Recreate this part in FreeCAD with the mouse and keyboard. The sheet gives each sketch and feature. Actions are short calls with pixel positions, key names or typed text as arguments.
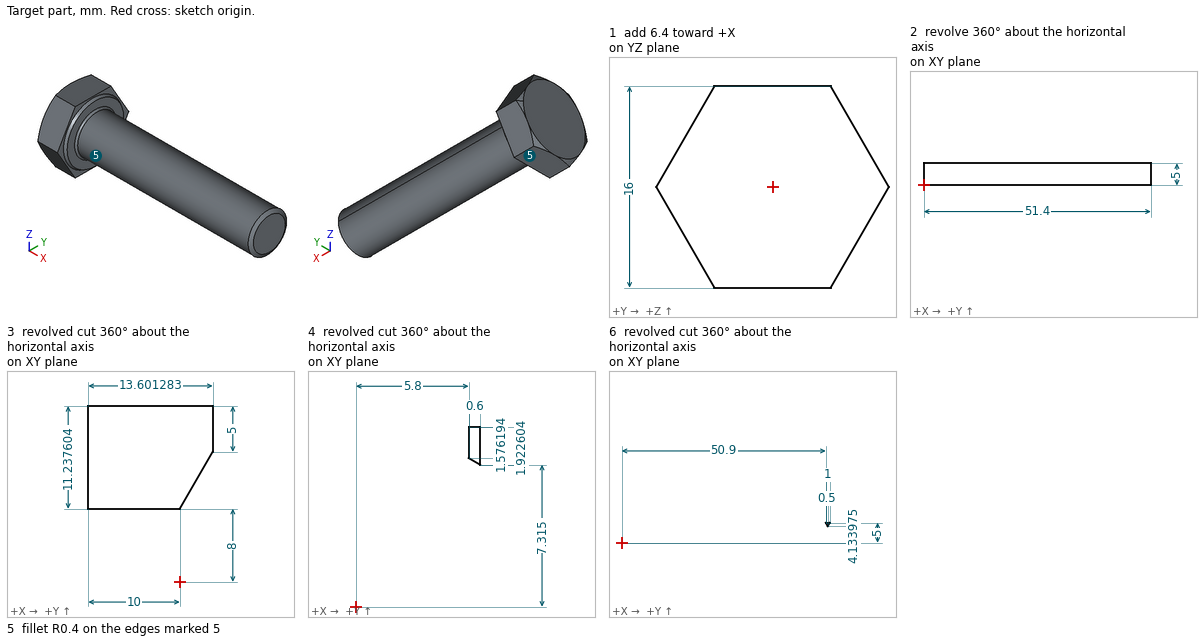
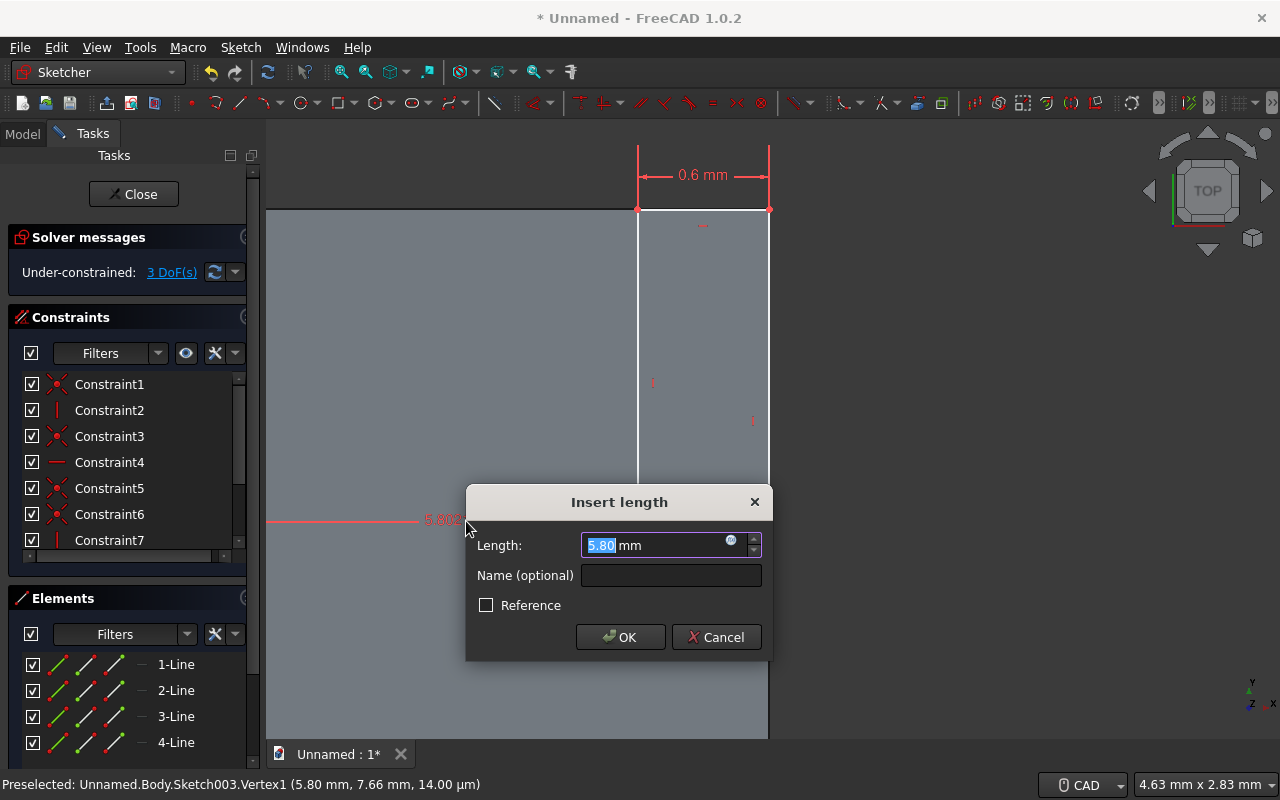
text(5.8)
key(Return)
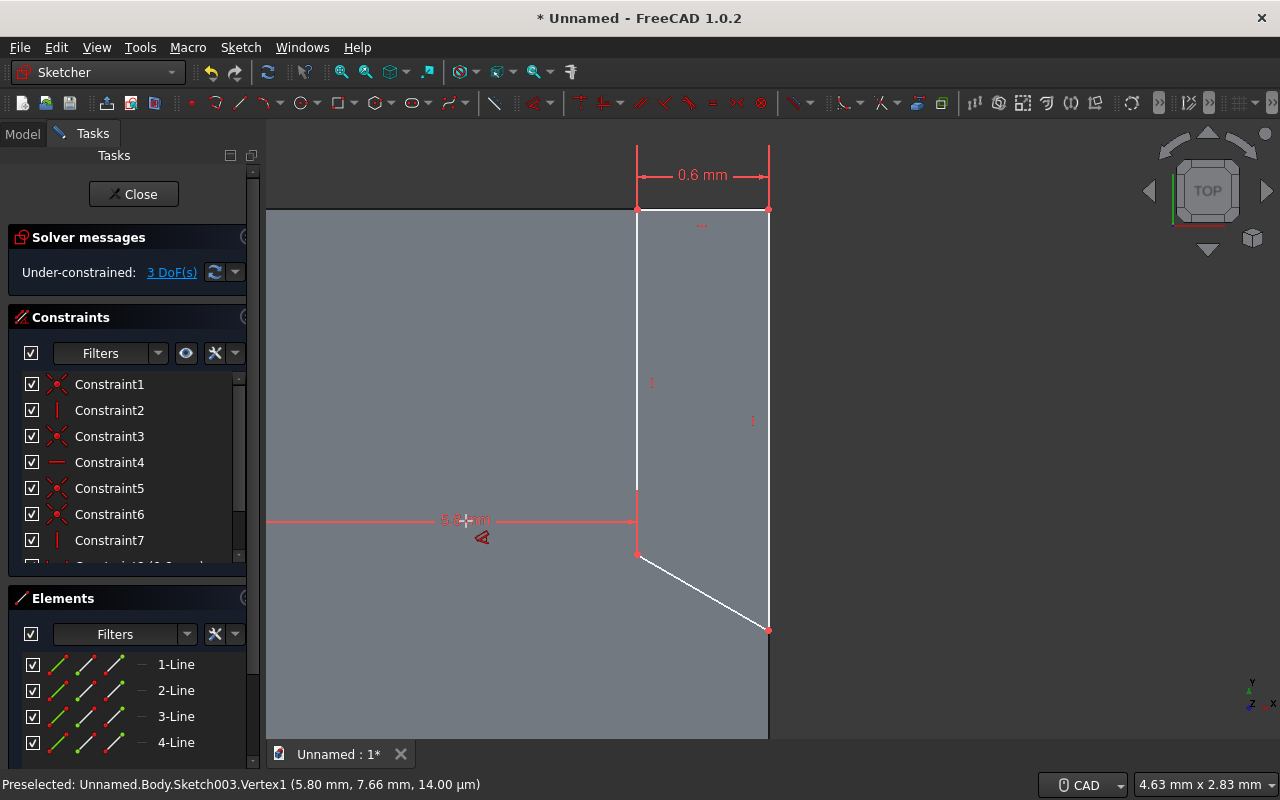
click(769, 631)
click(803, 671)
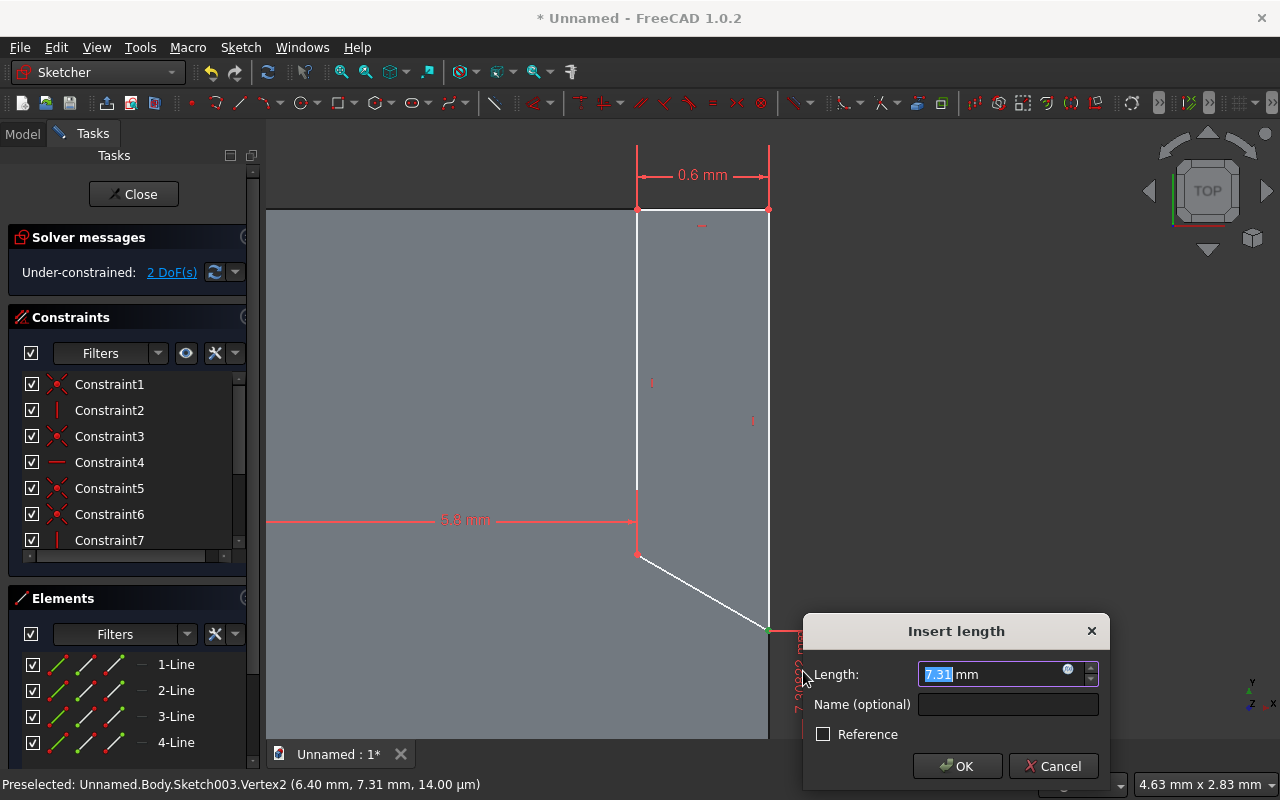
text(7.315)
key(Return)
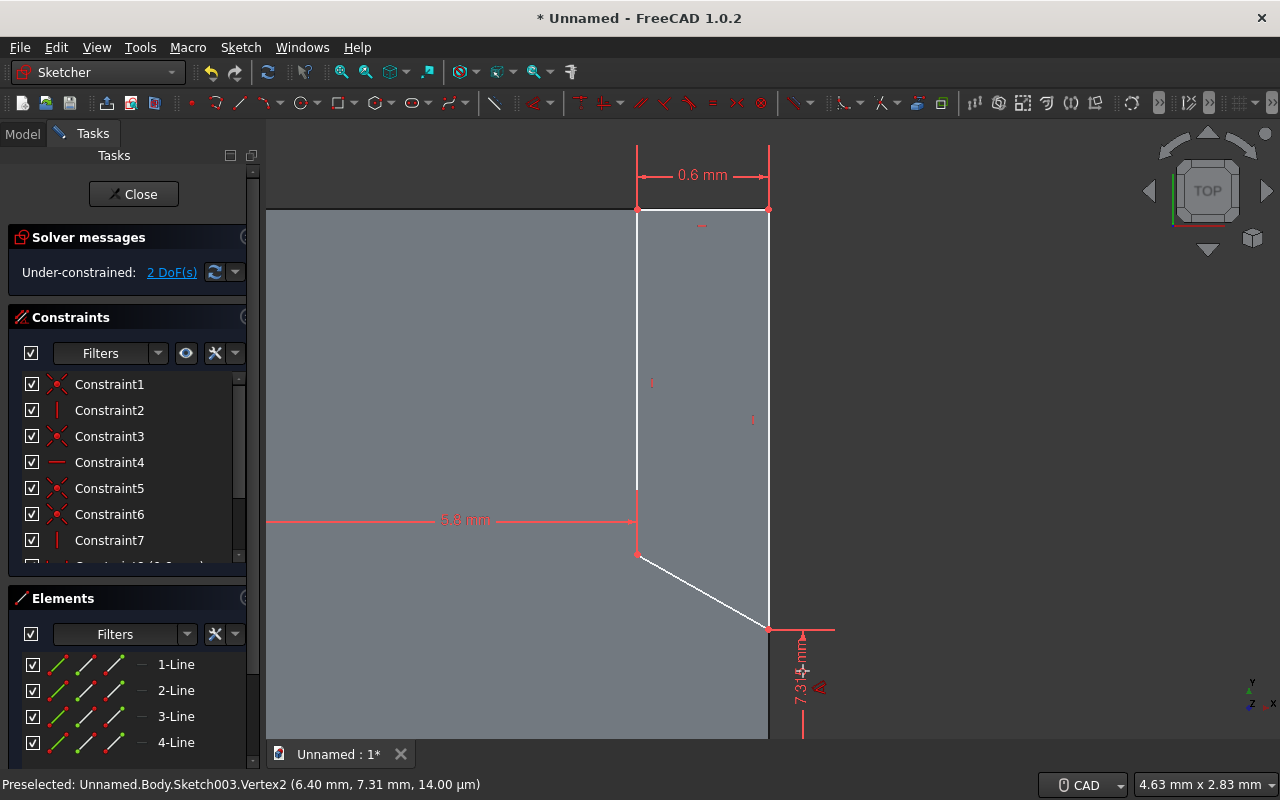
click(769, 504)
click(803, 420)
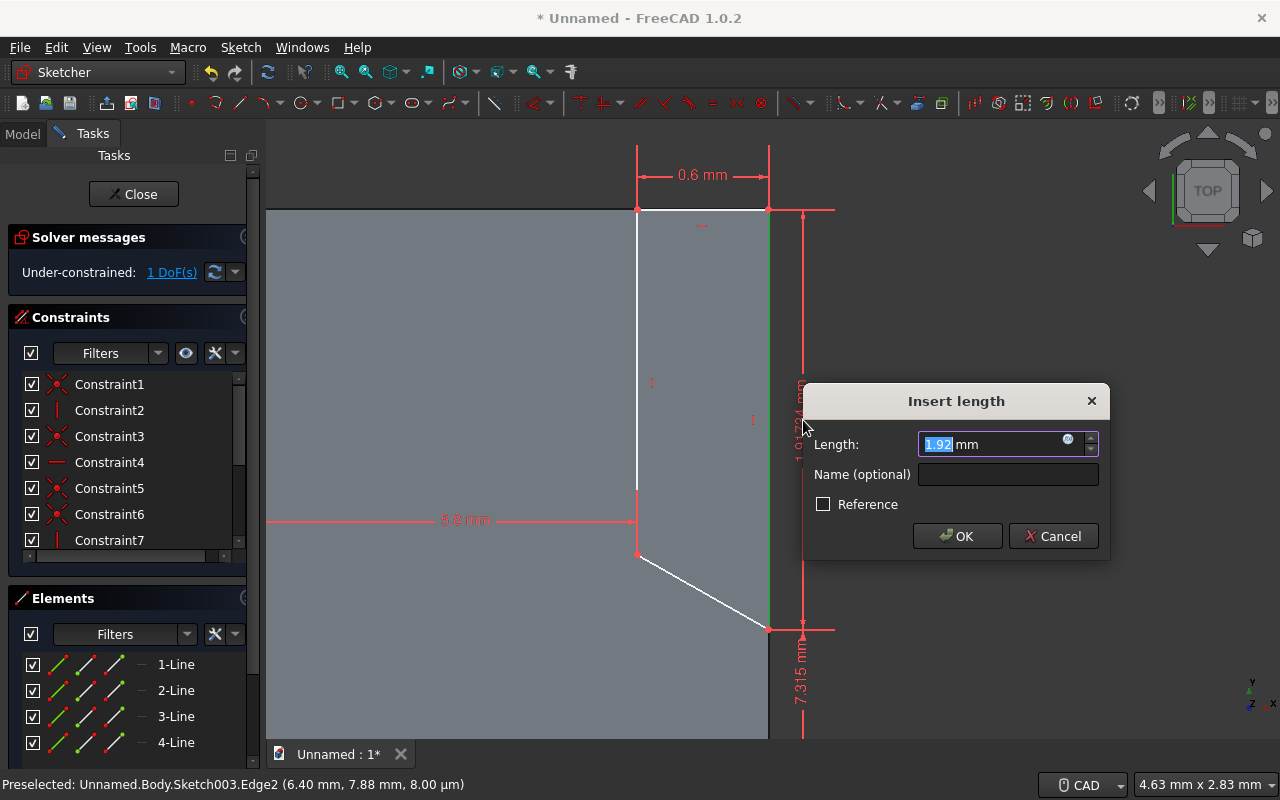
text(1.922604)
key(Return)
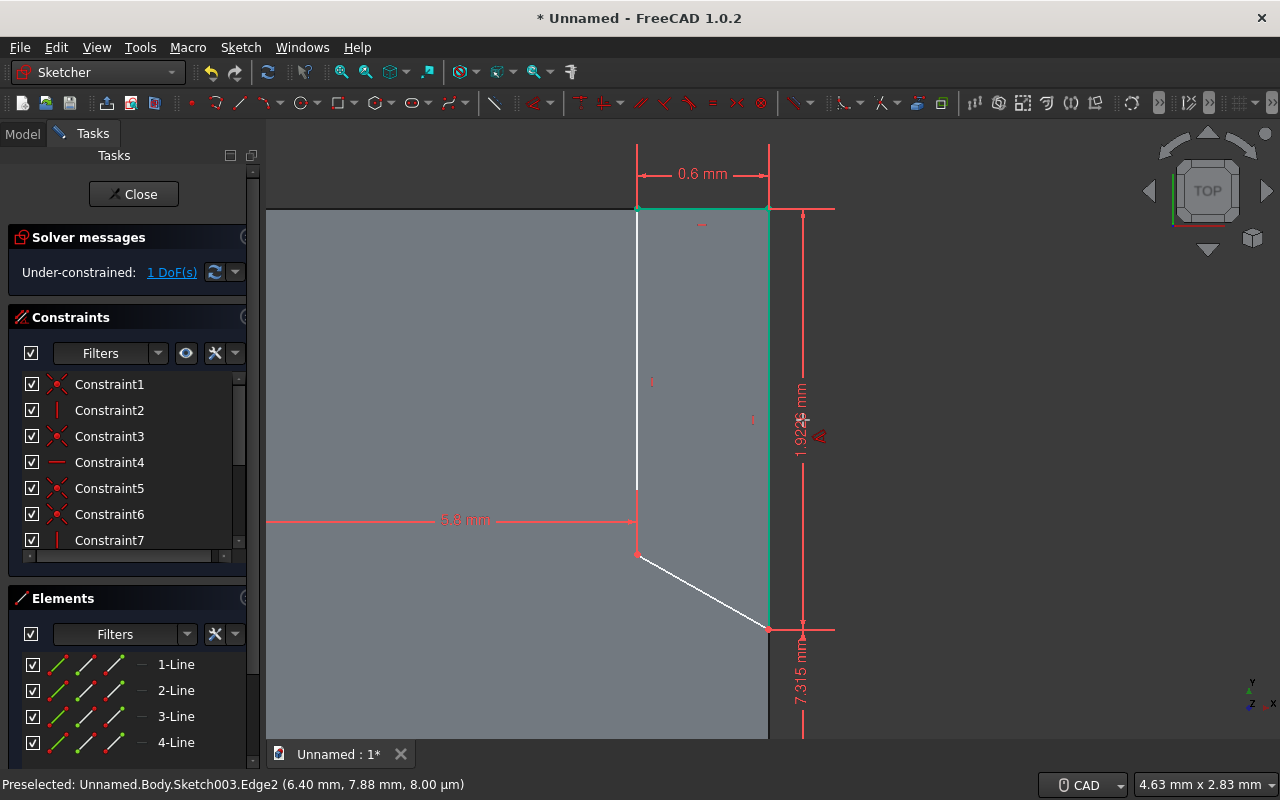
click(637, 313)
click(603, 382)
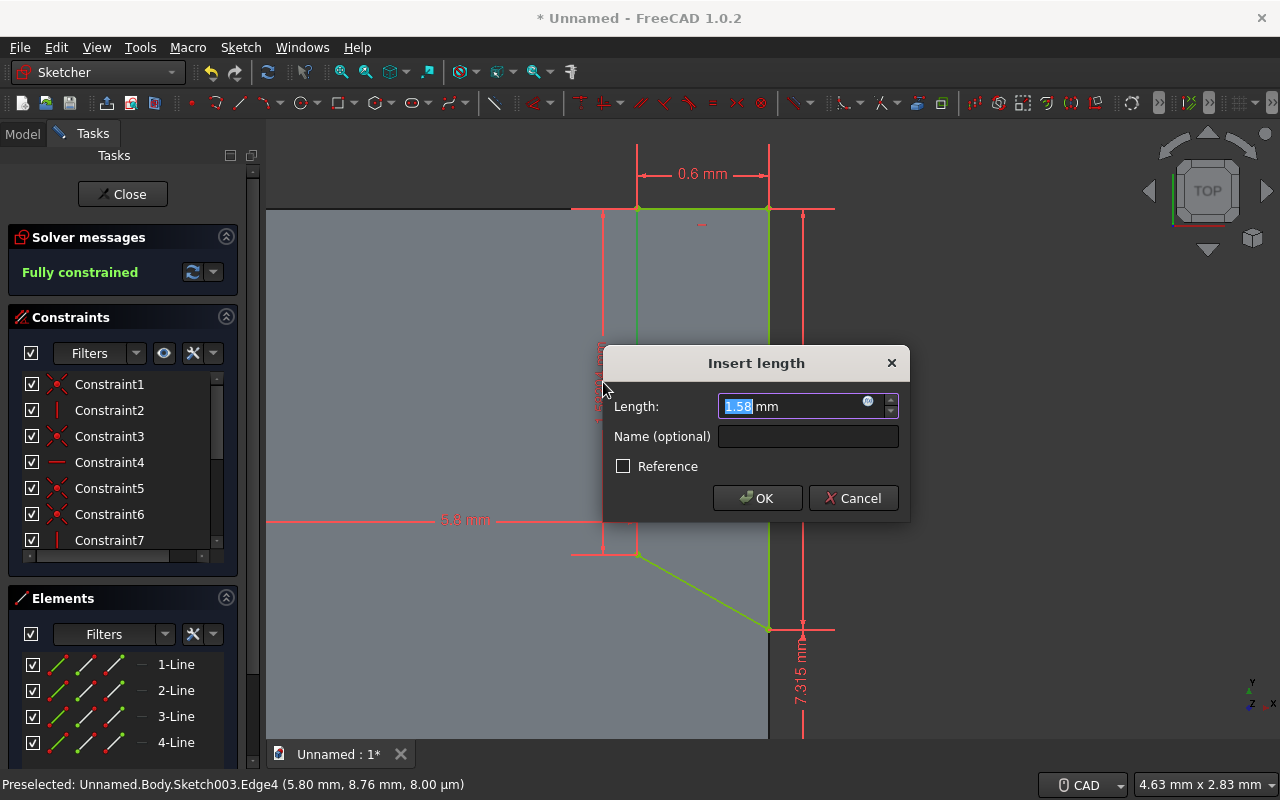
text(1.576194)
key(Return)
key(Escape)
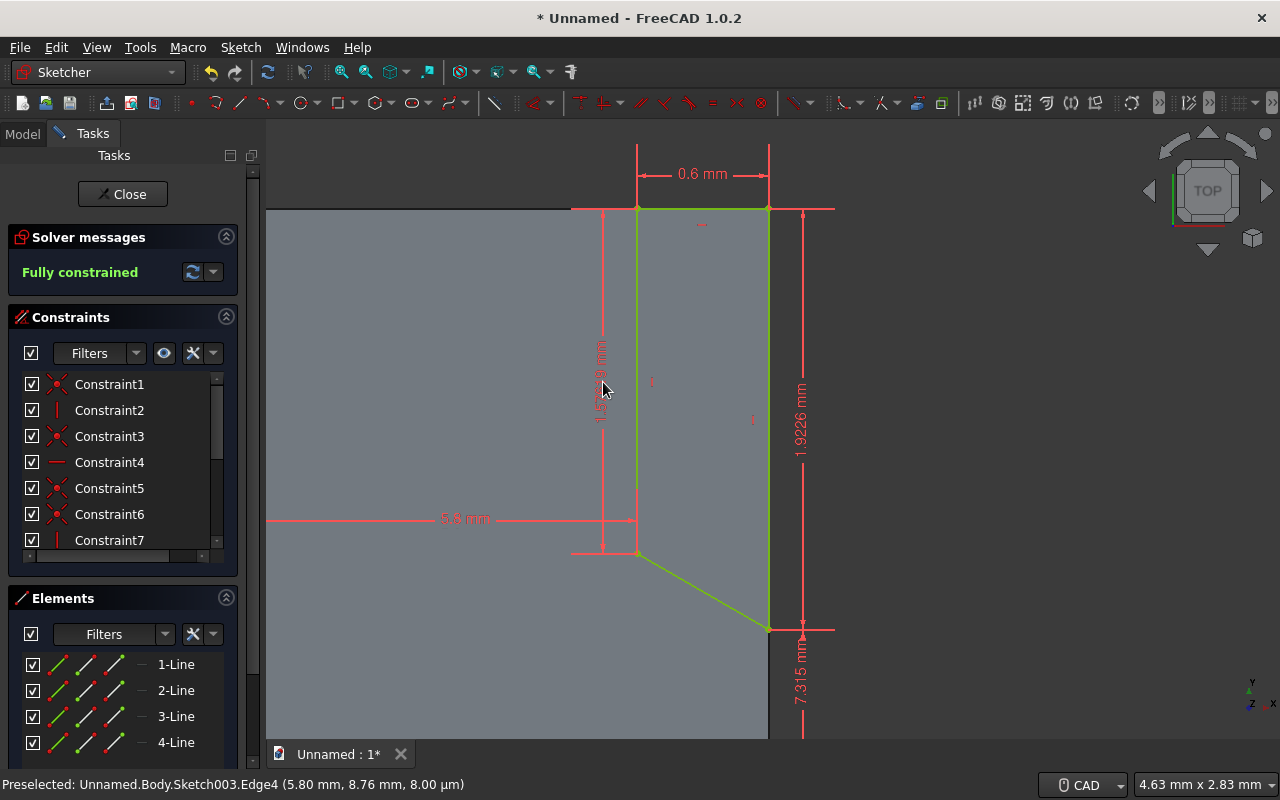
click(123, 194)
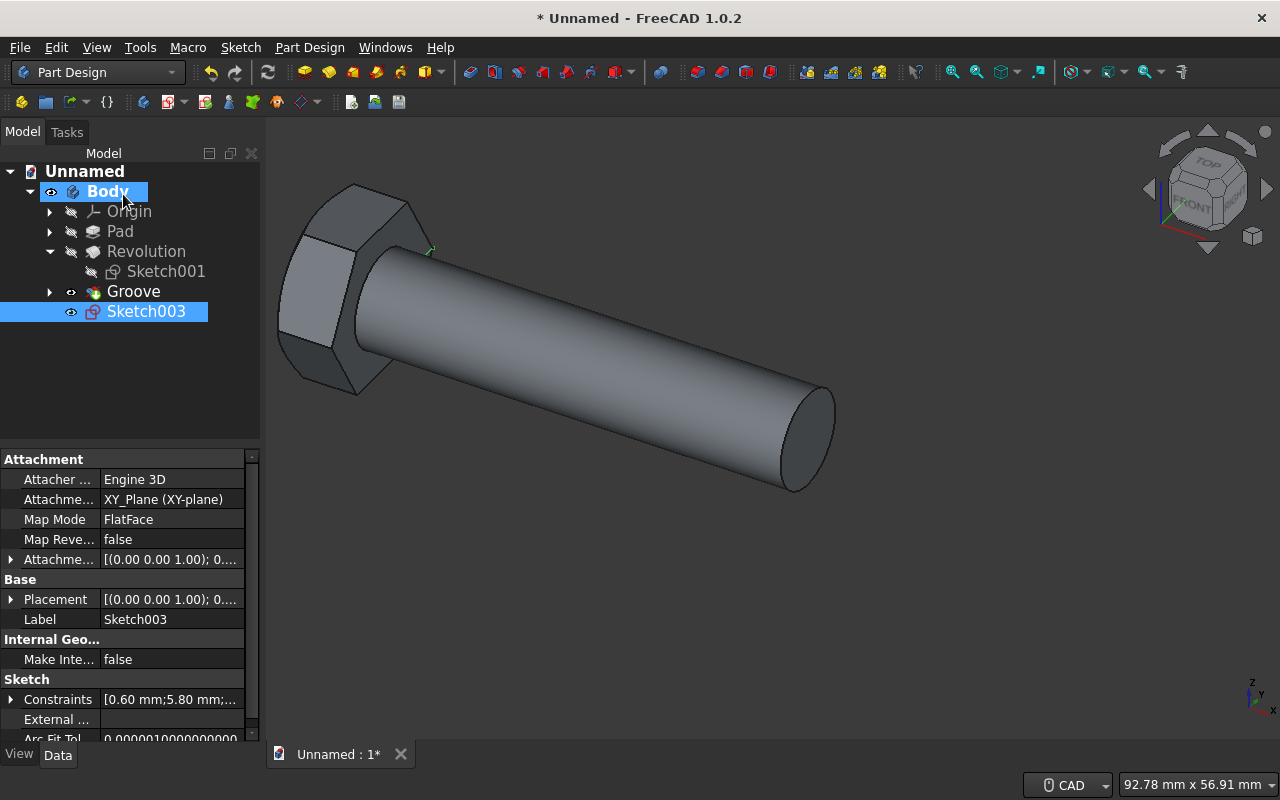
click(520, 72)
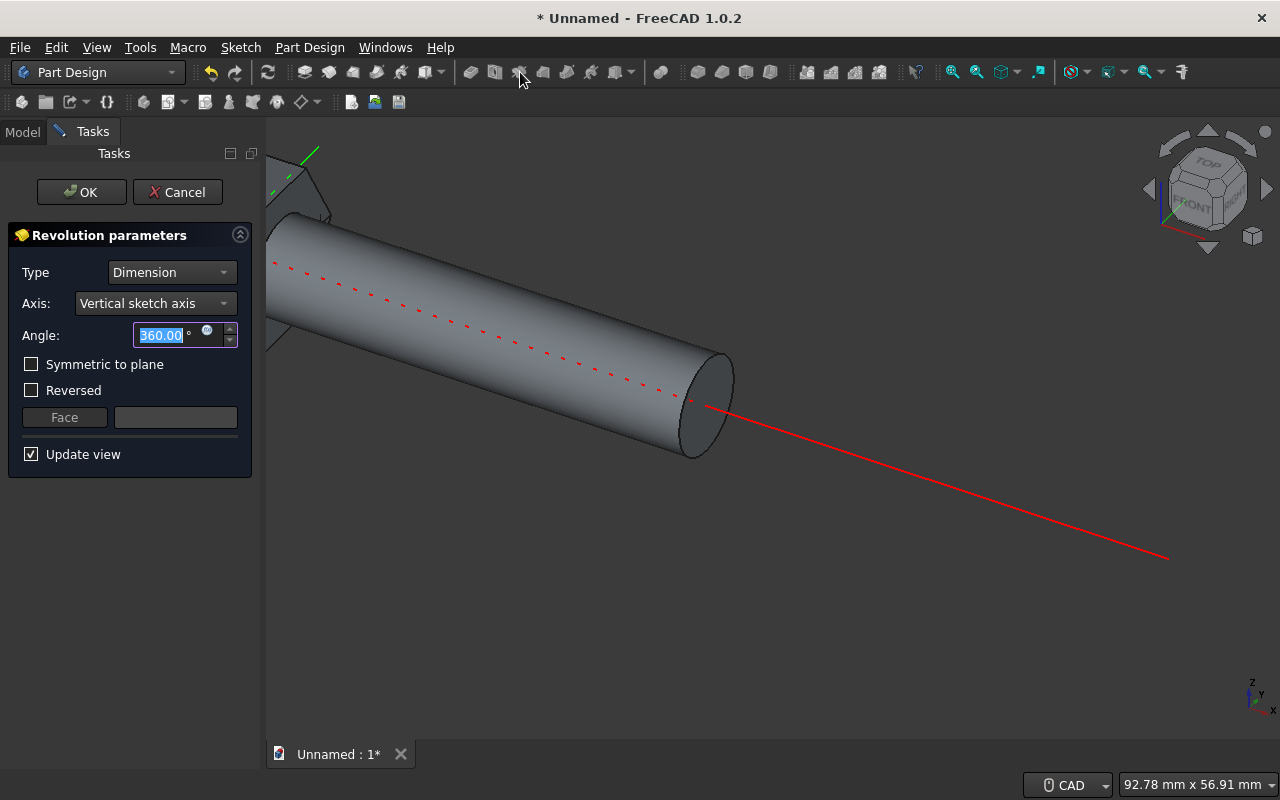
click(156, 304)